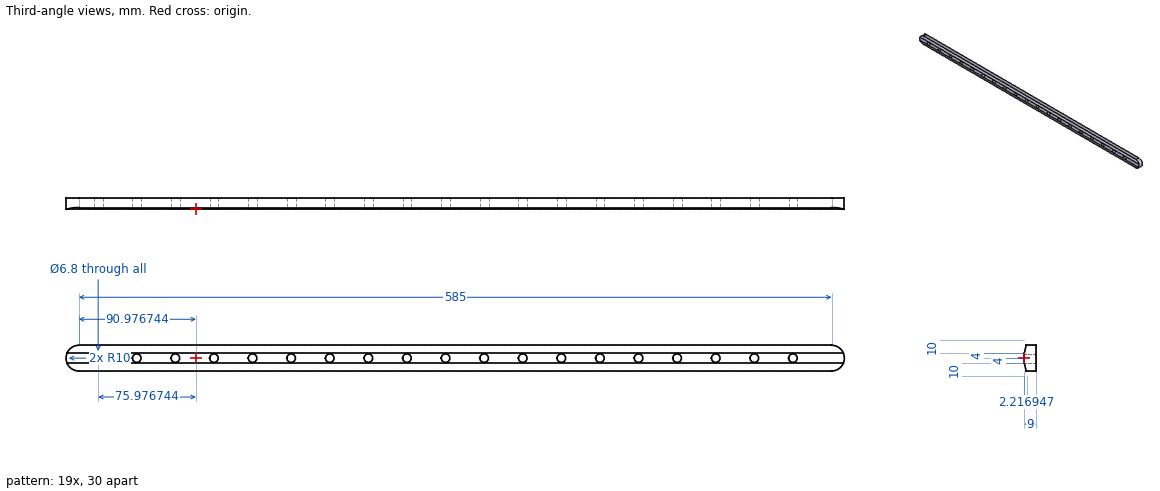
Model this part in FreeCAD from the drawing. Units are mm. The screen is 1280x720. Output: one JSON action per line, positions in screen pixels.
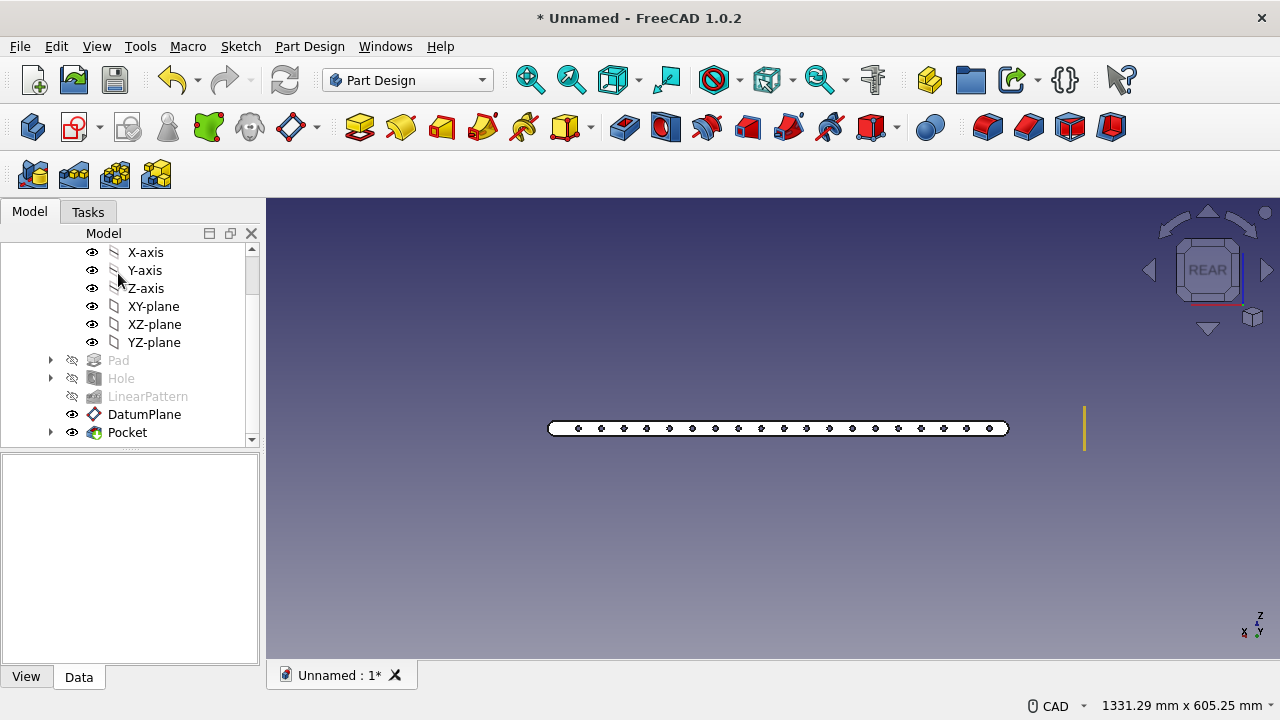
{"action": "left_click", "coordinate": [117, 414]}
{"action": "key", "text": "space"}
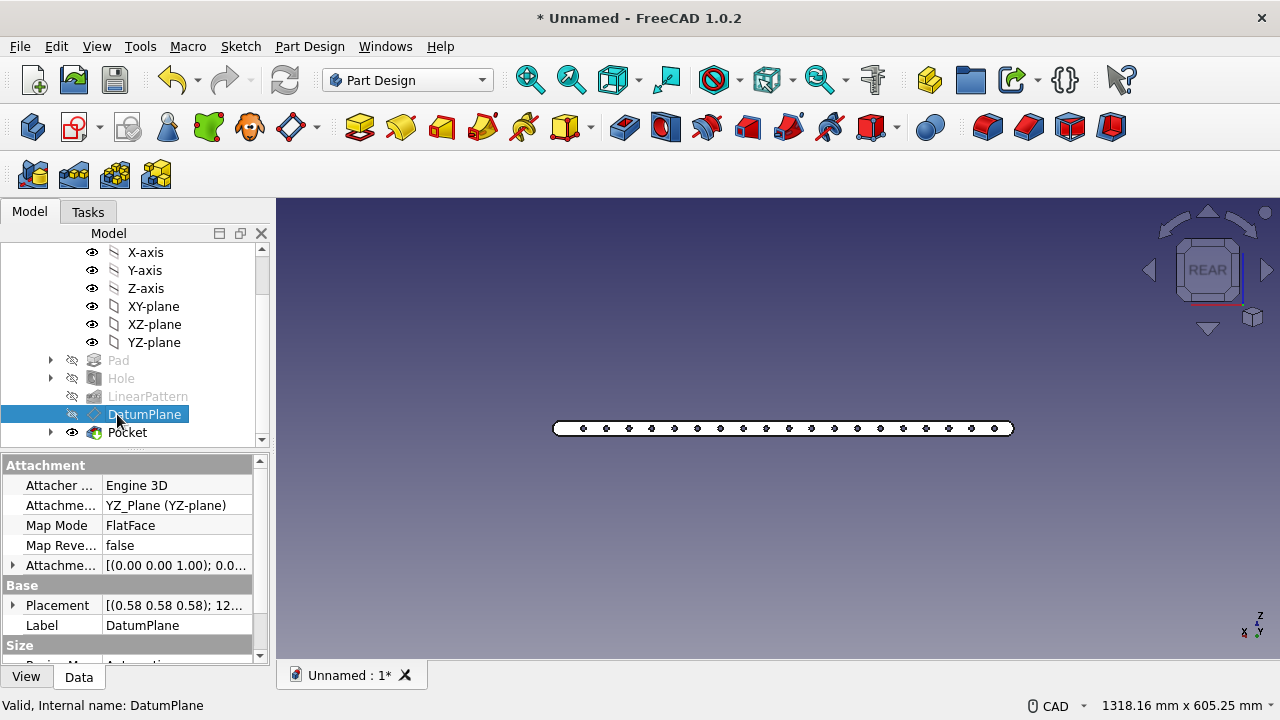
{"action": "key", "text": "0"}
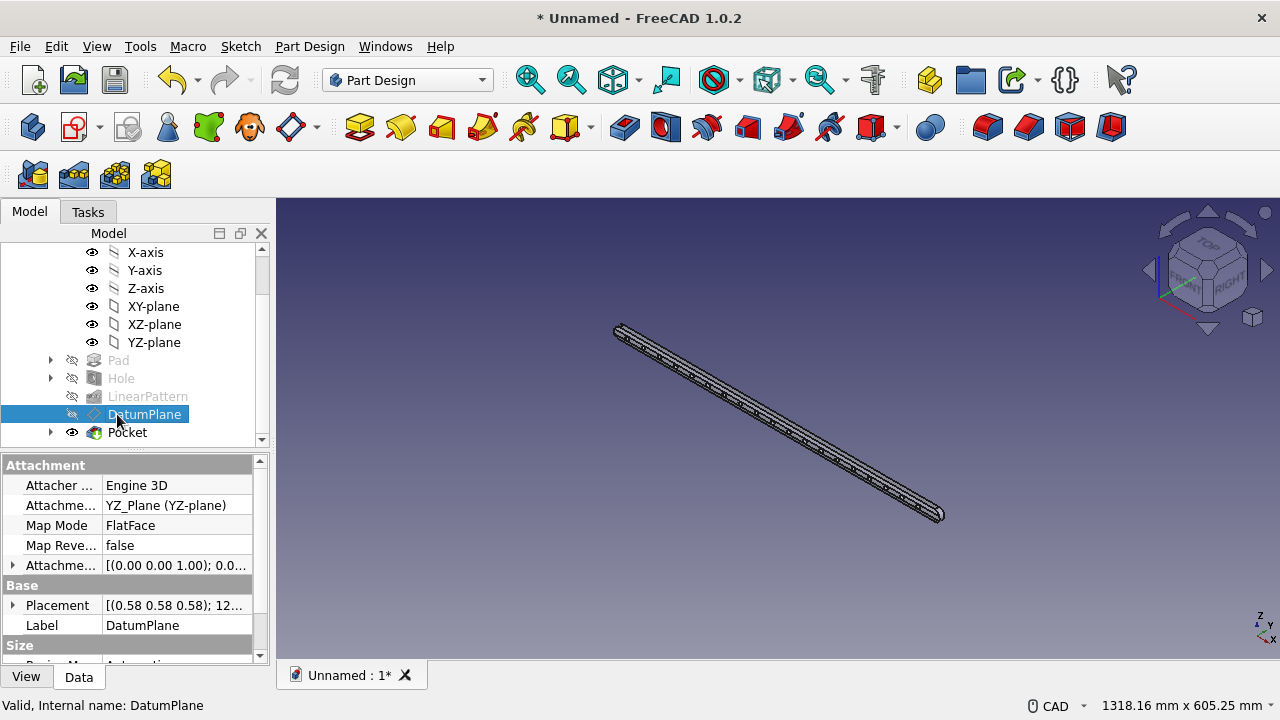
{"action": "left_click", "coordinate": [531, 80]}